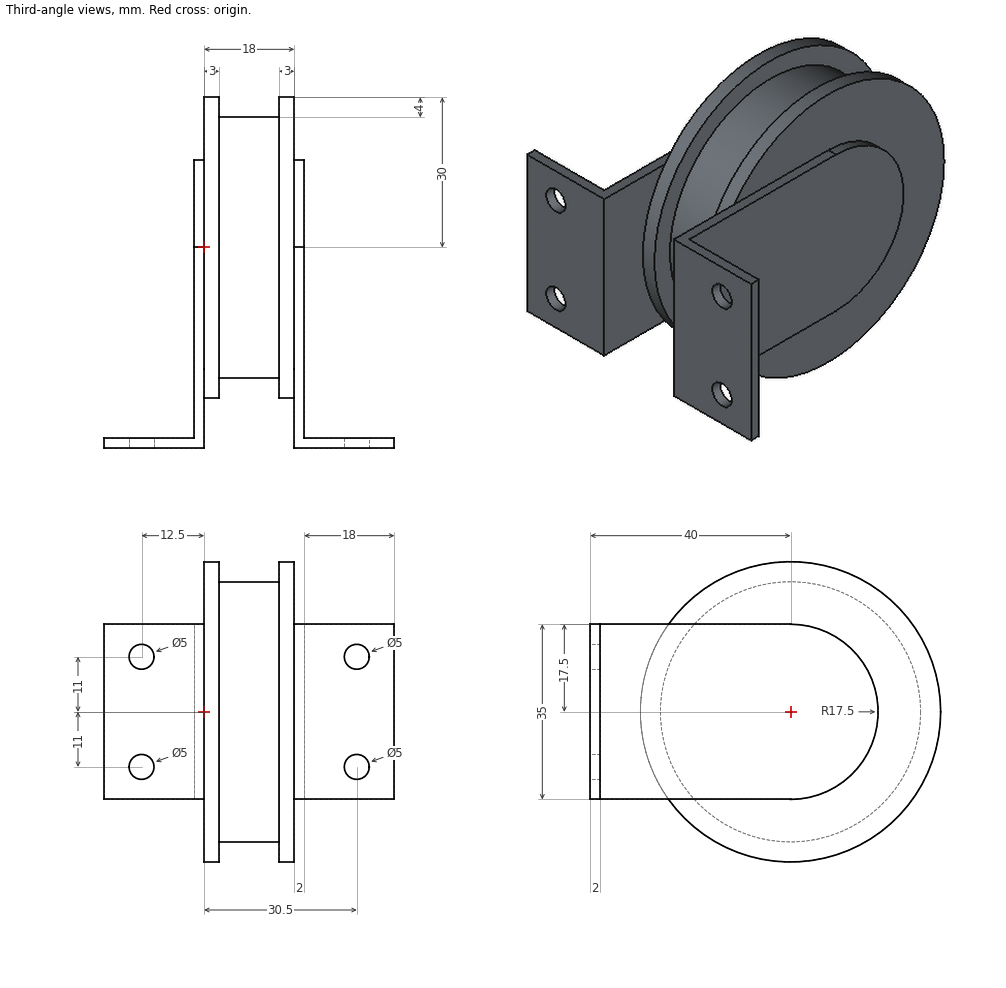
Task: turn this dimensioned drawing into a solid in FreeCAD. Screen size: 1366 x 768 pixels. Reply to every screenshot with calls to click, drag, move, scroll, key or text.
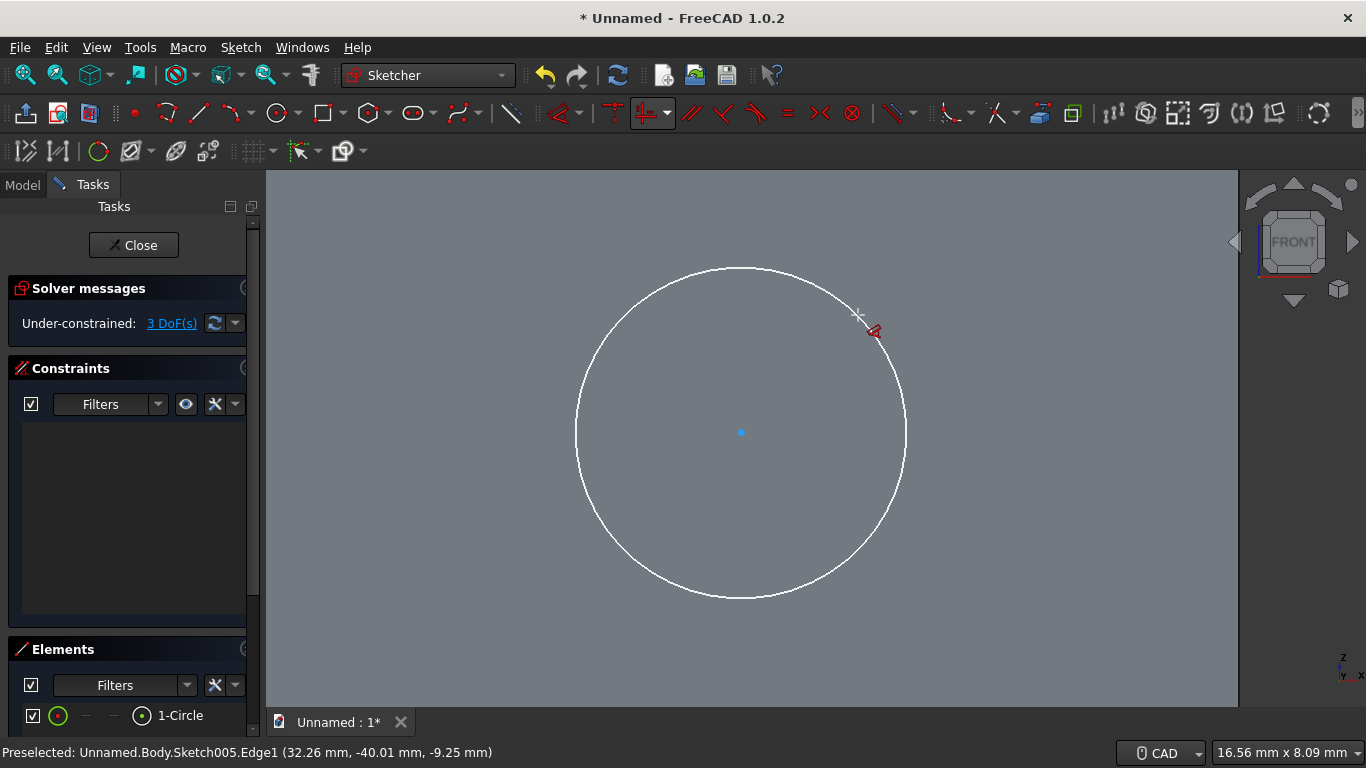
click(858, 316)
click(881, 293)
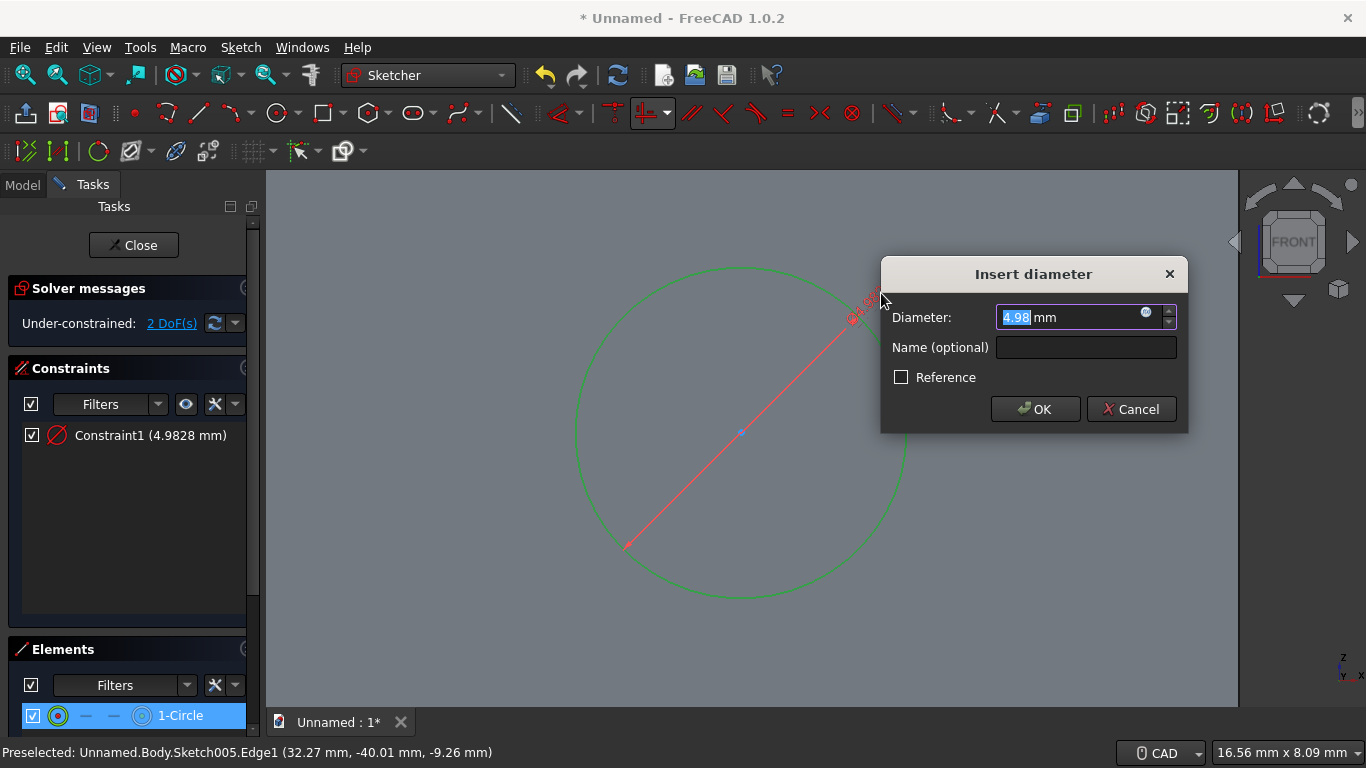
text(5)
key(Return)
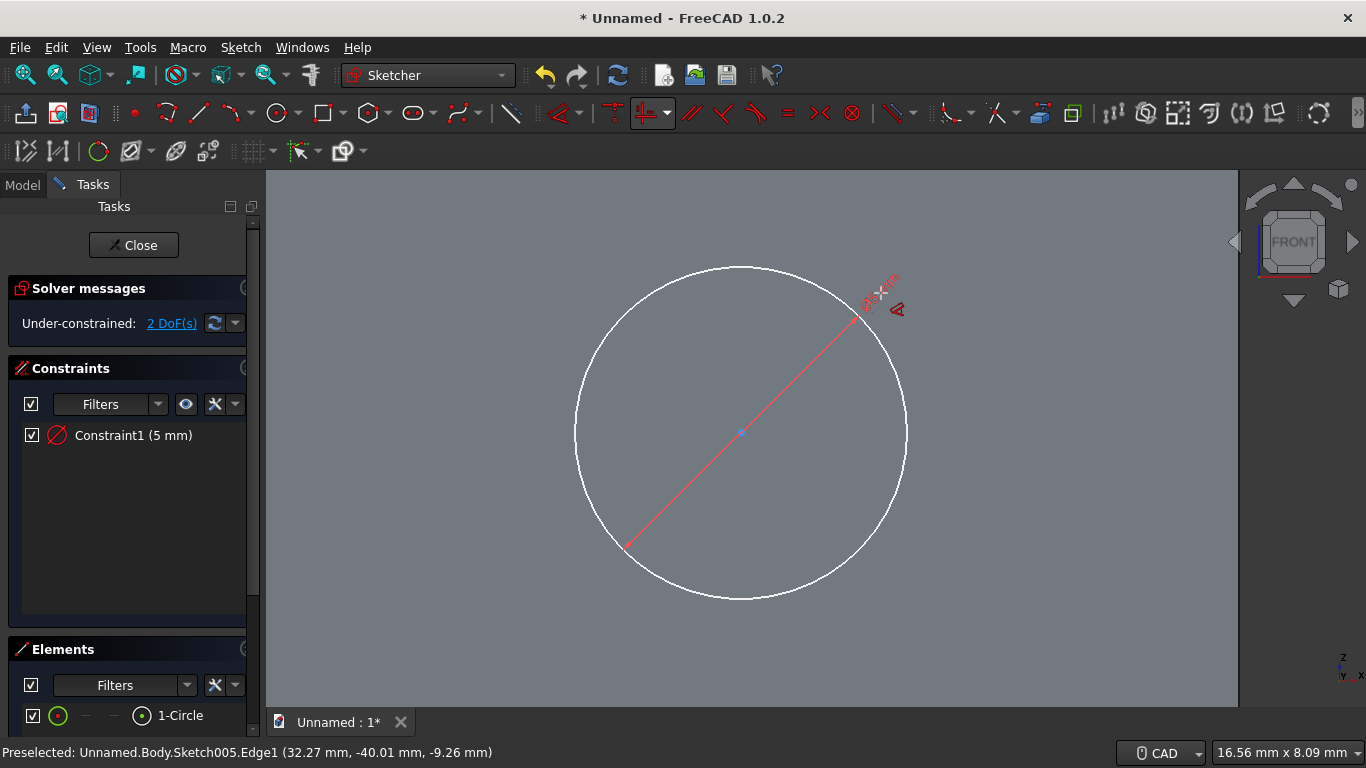
click(741, 433)
click(775, 315)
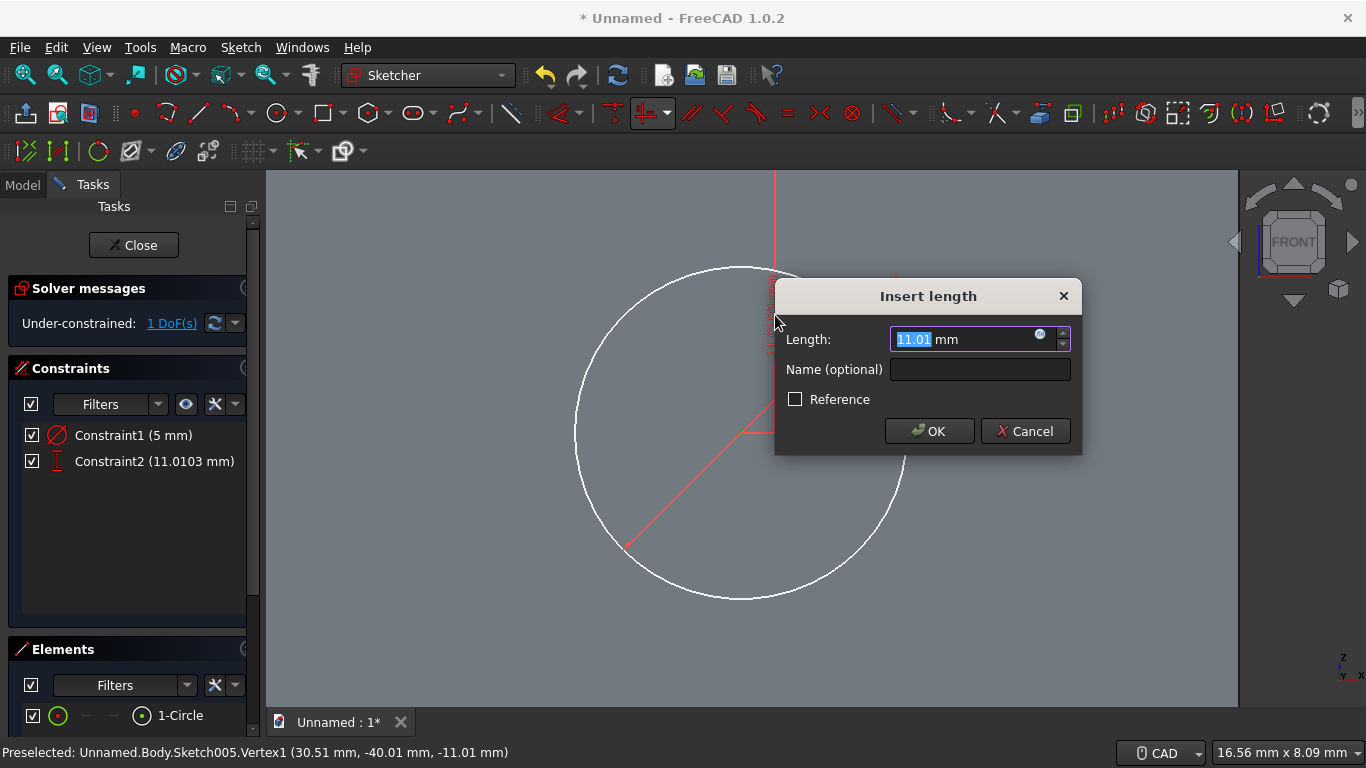
text(11)
key(Return)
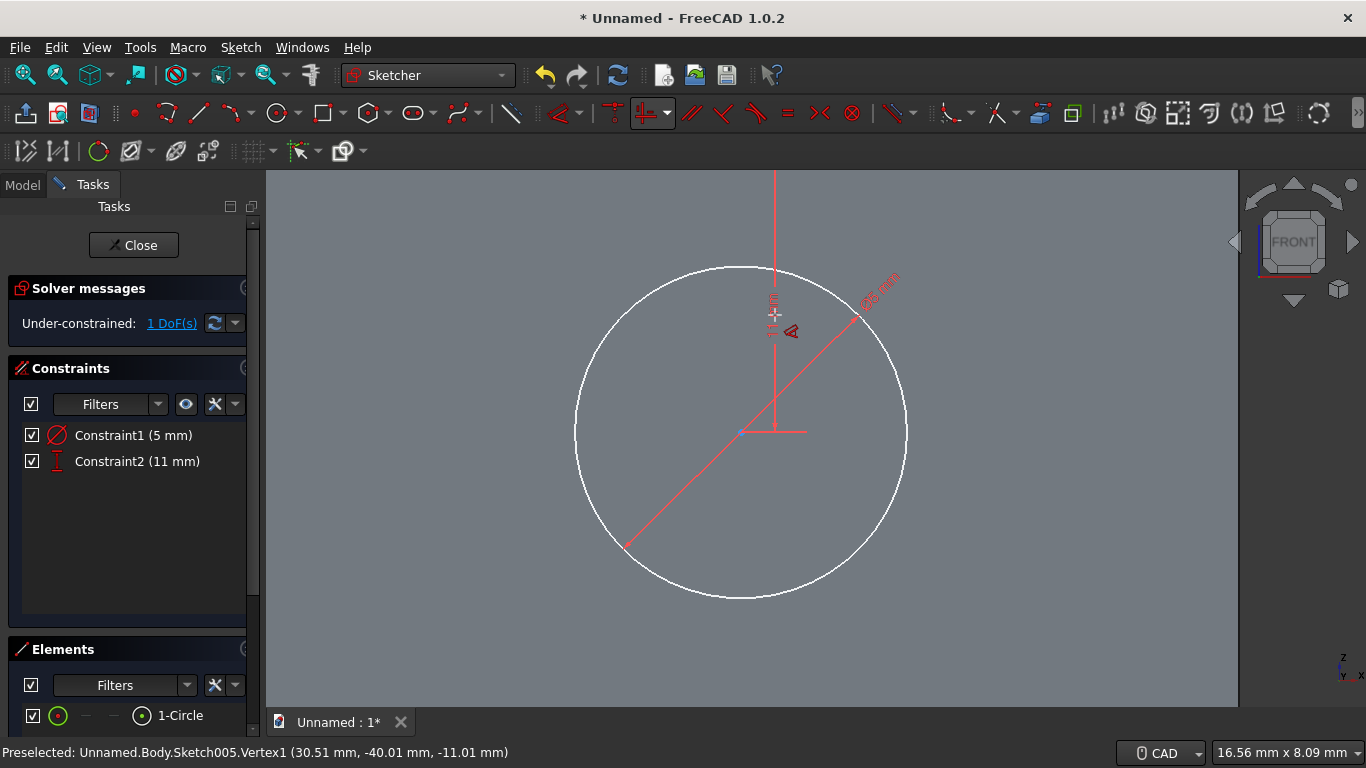
click(741, 432)
click(518, 466)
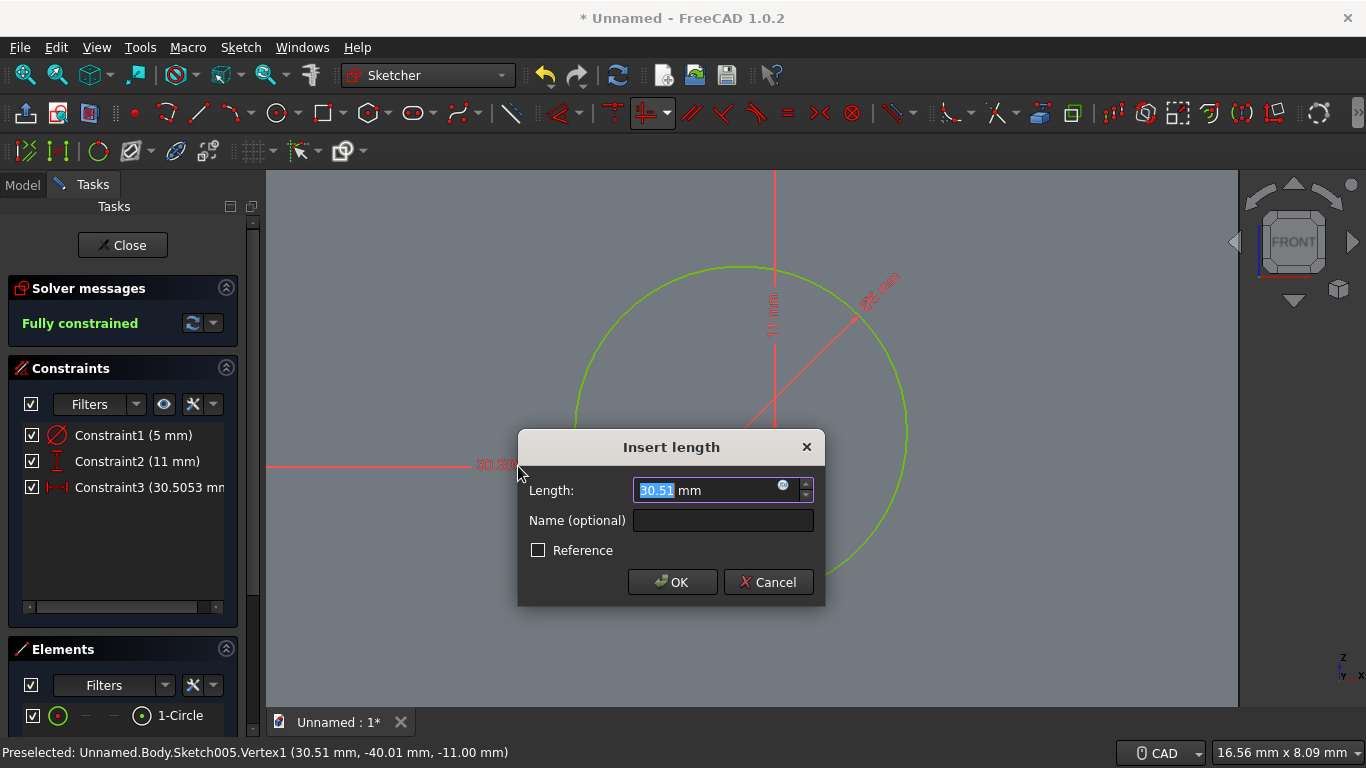
text(30.5)
key(Return)
key(Escape)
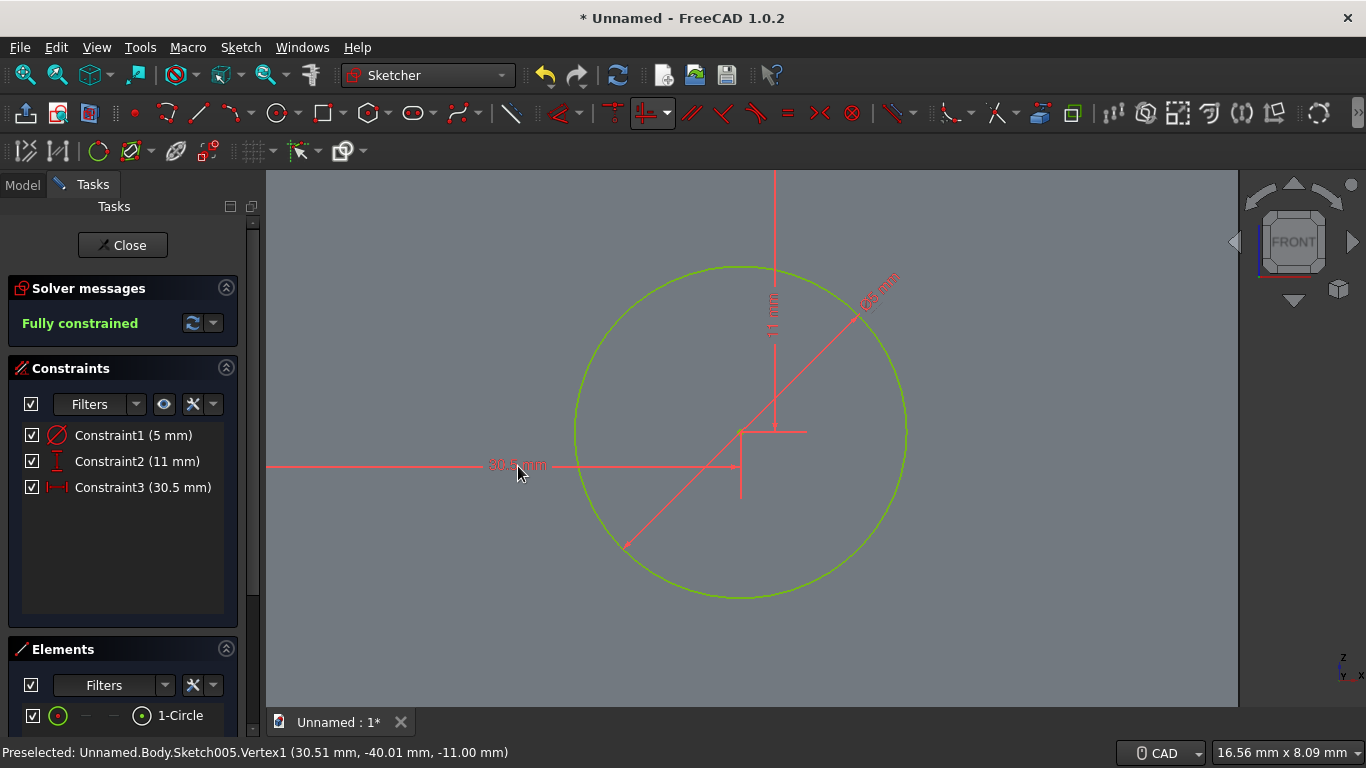
click(123, 245)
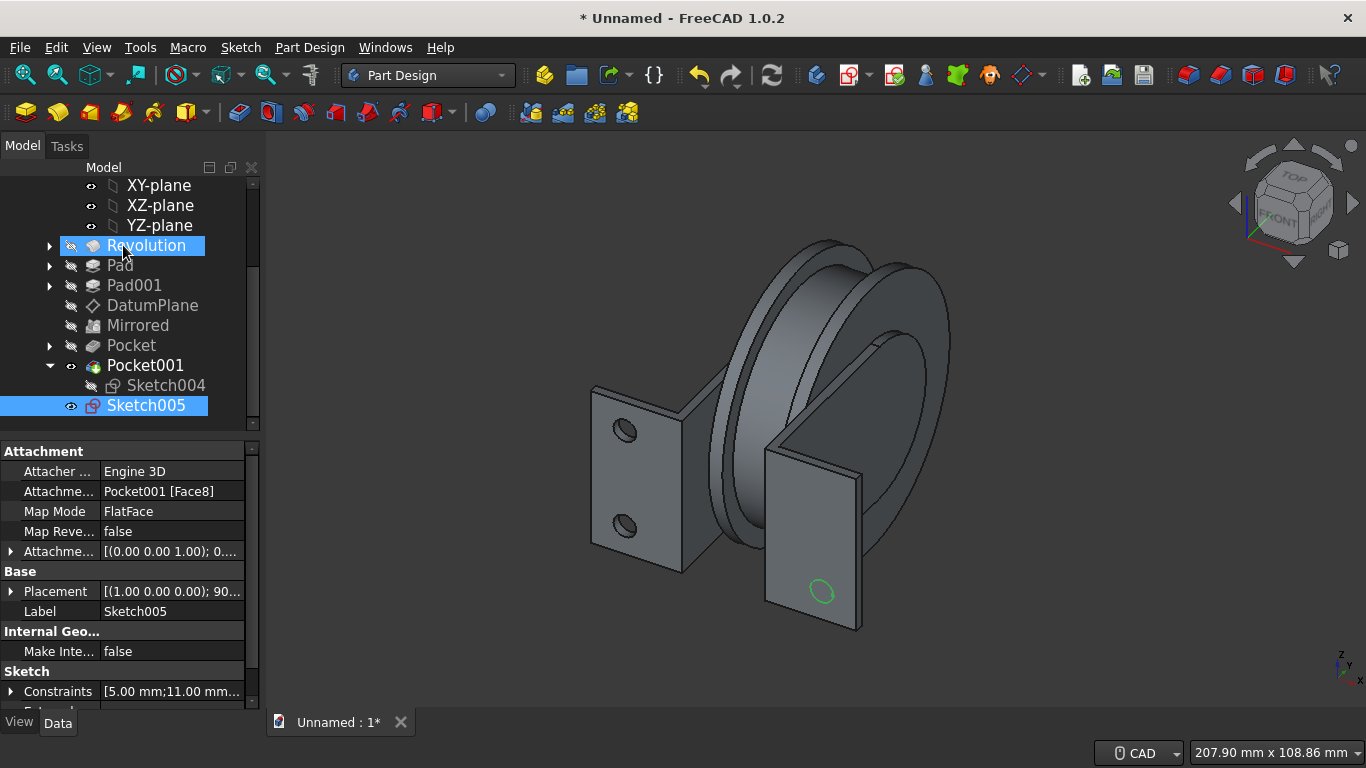
click(240, 112)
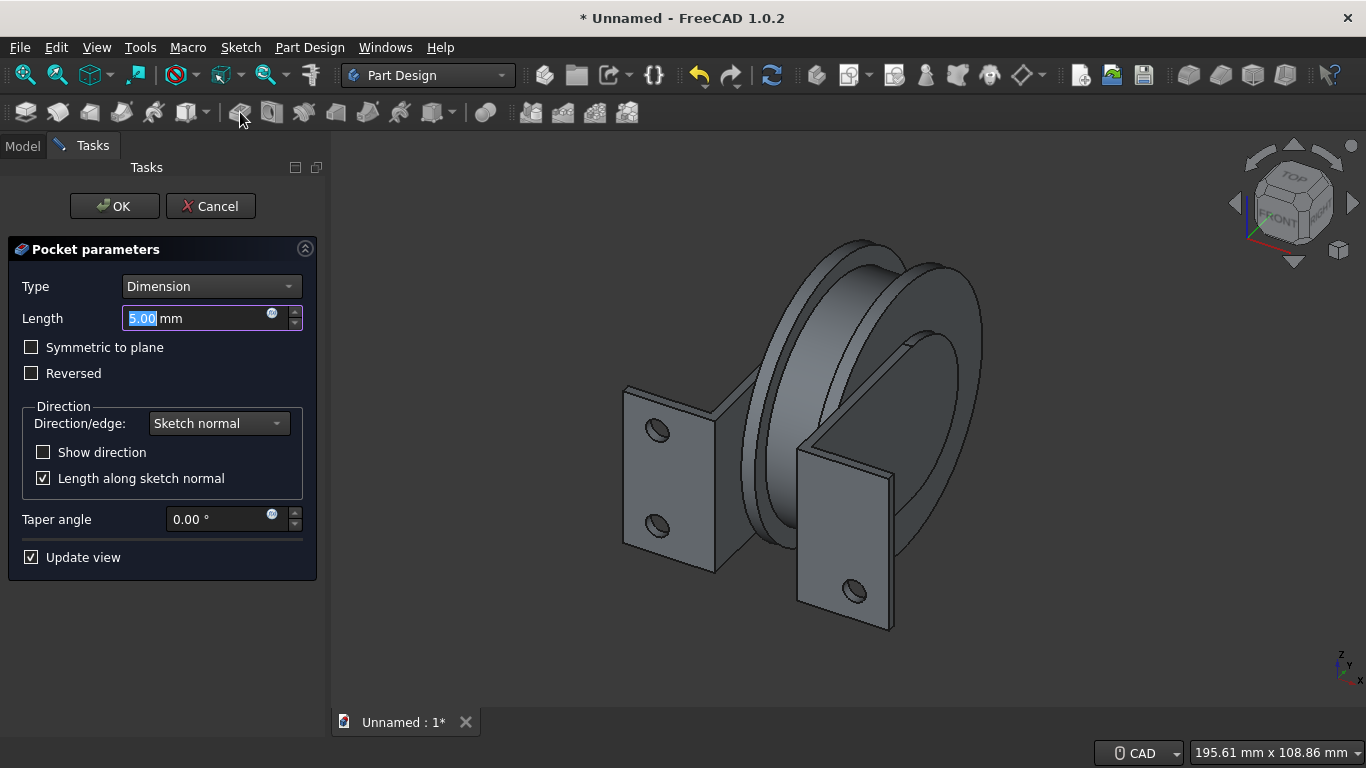
click(212, 286)